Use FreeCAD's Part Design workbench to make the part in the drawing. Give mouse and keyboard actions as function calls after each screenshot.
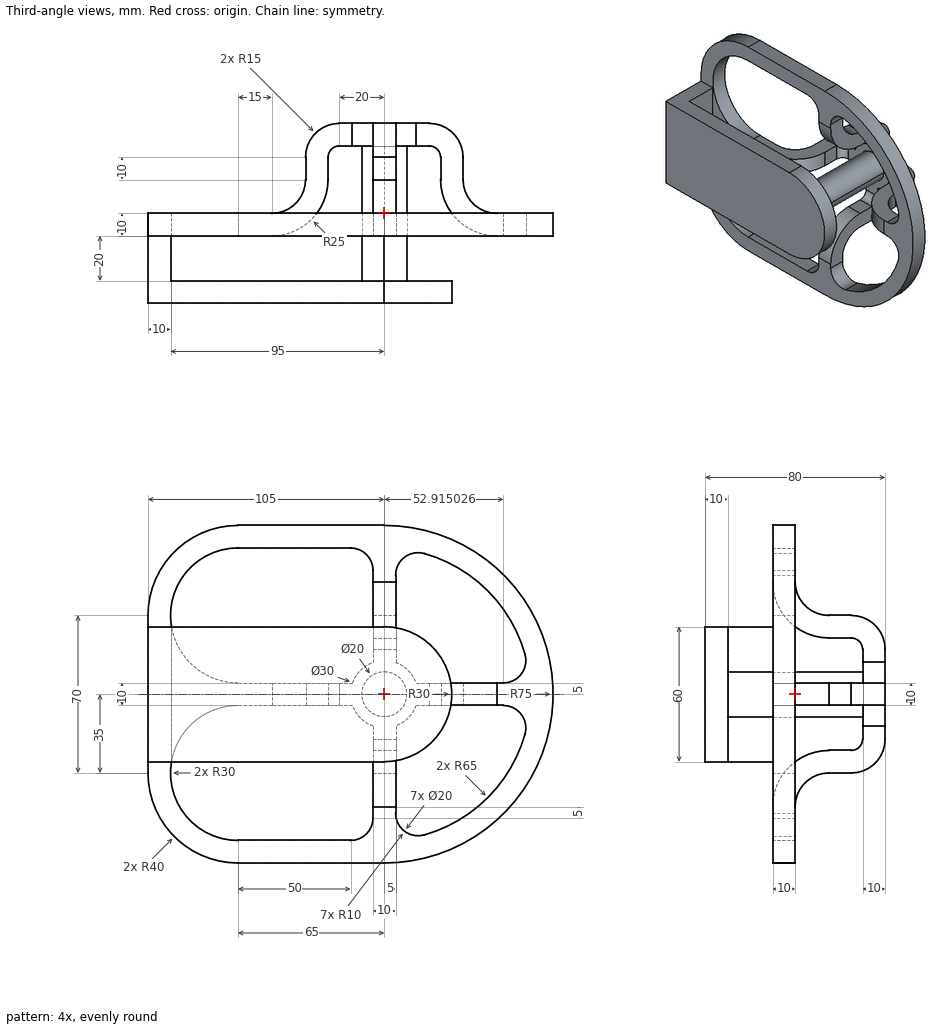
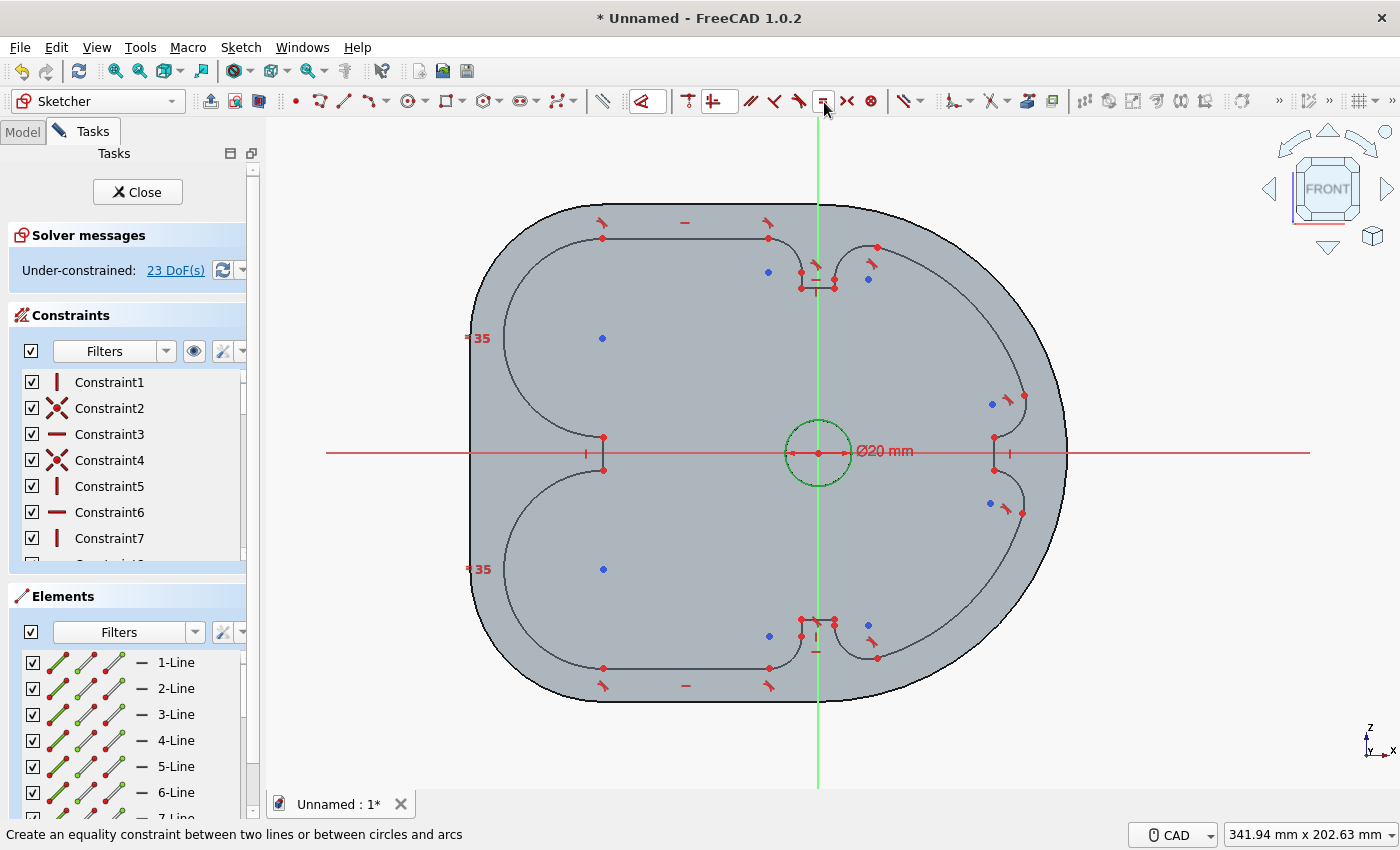
click(784, 665)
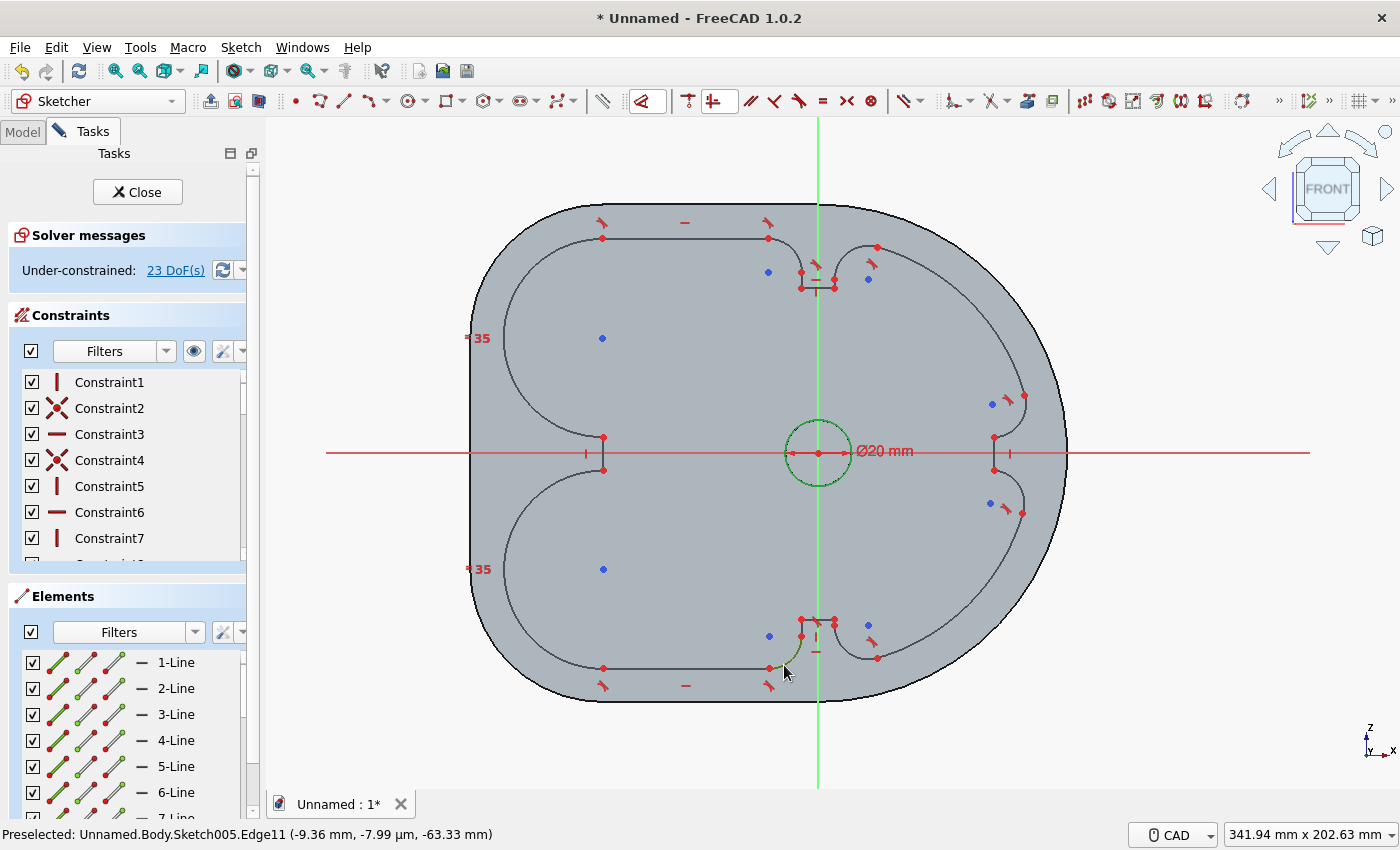
click(798, 257)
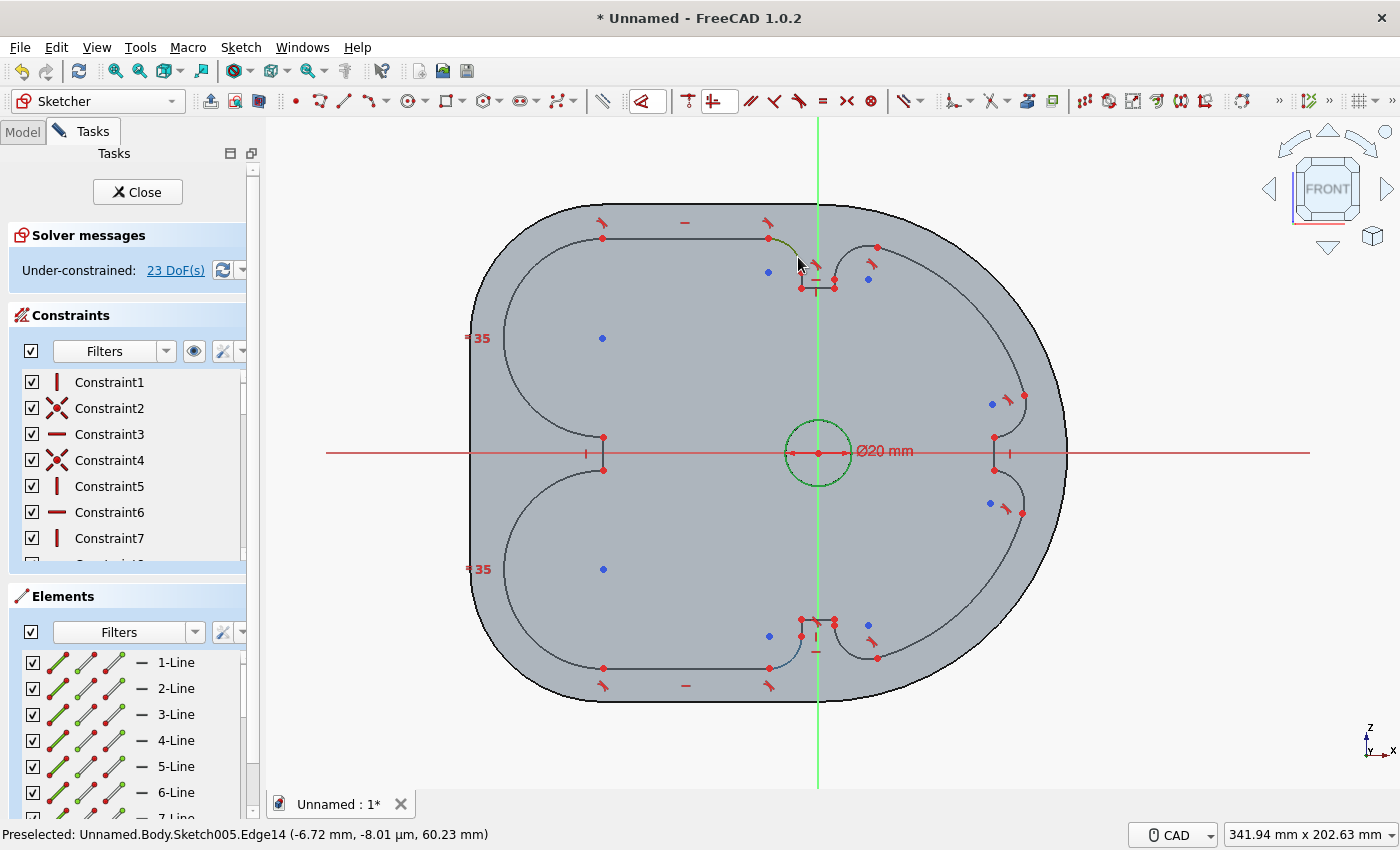
click(859, 247)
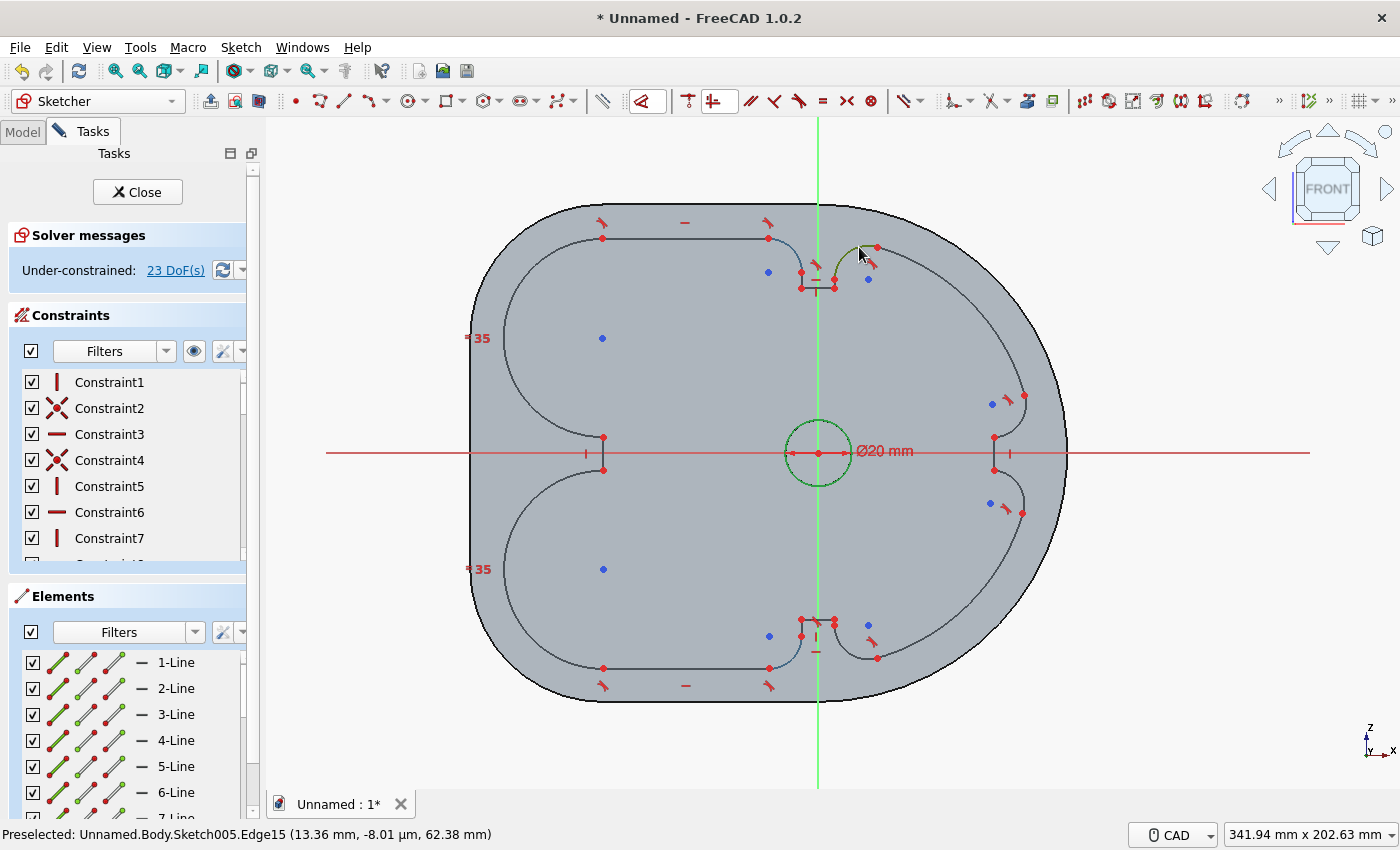
click(1011, 432)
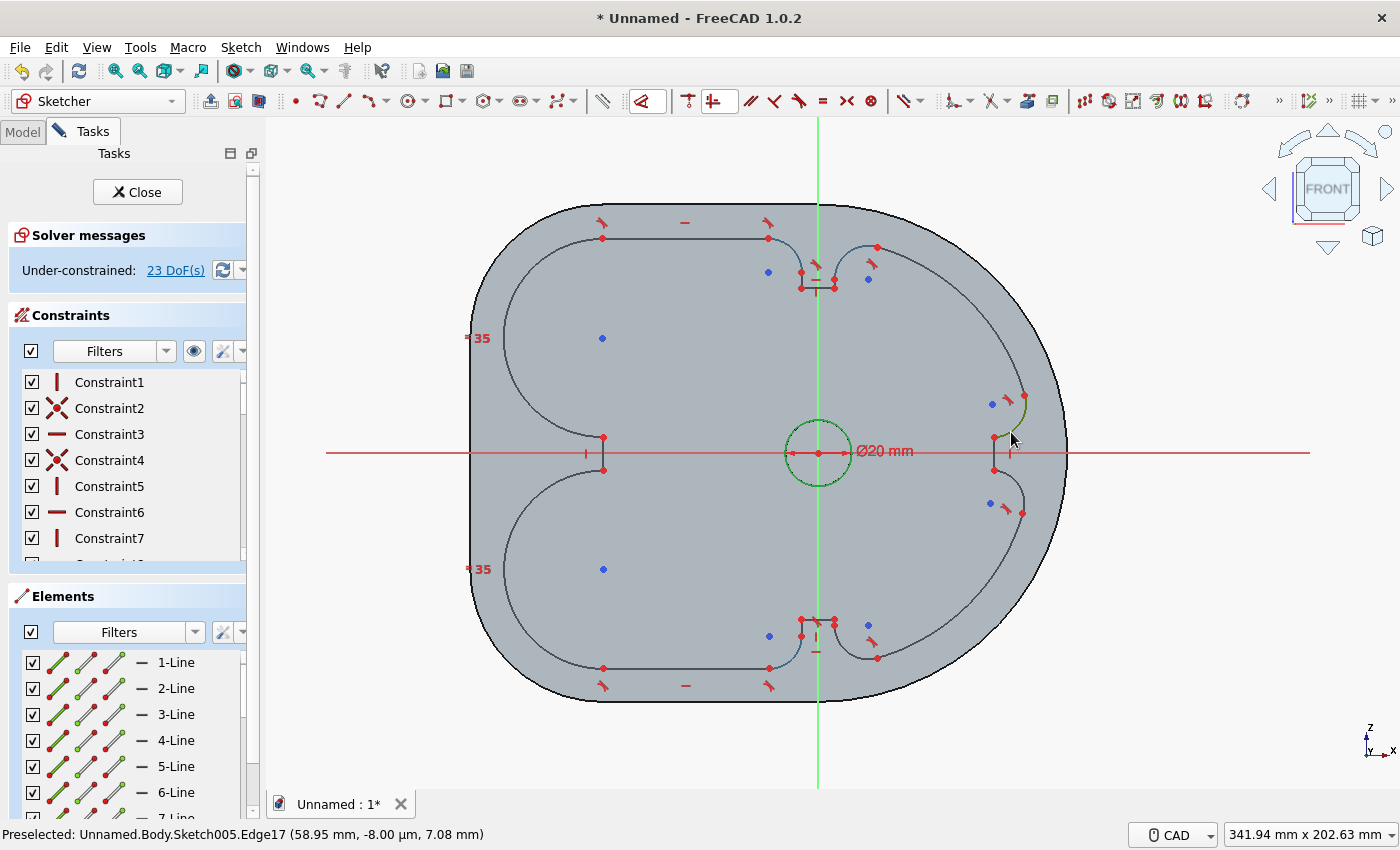
click(1023, 496)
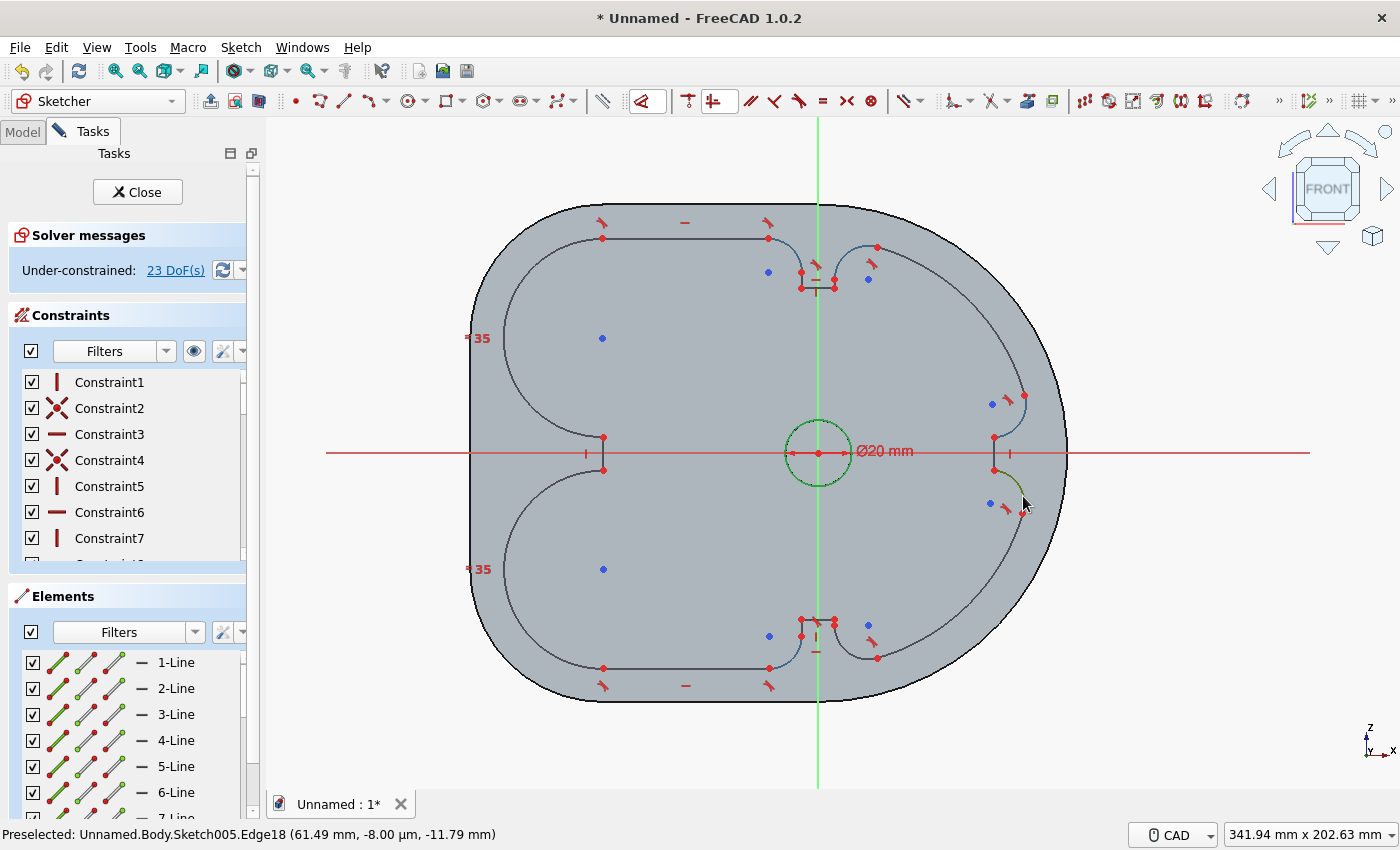
click(840, 644)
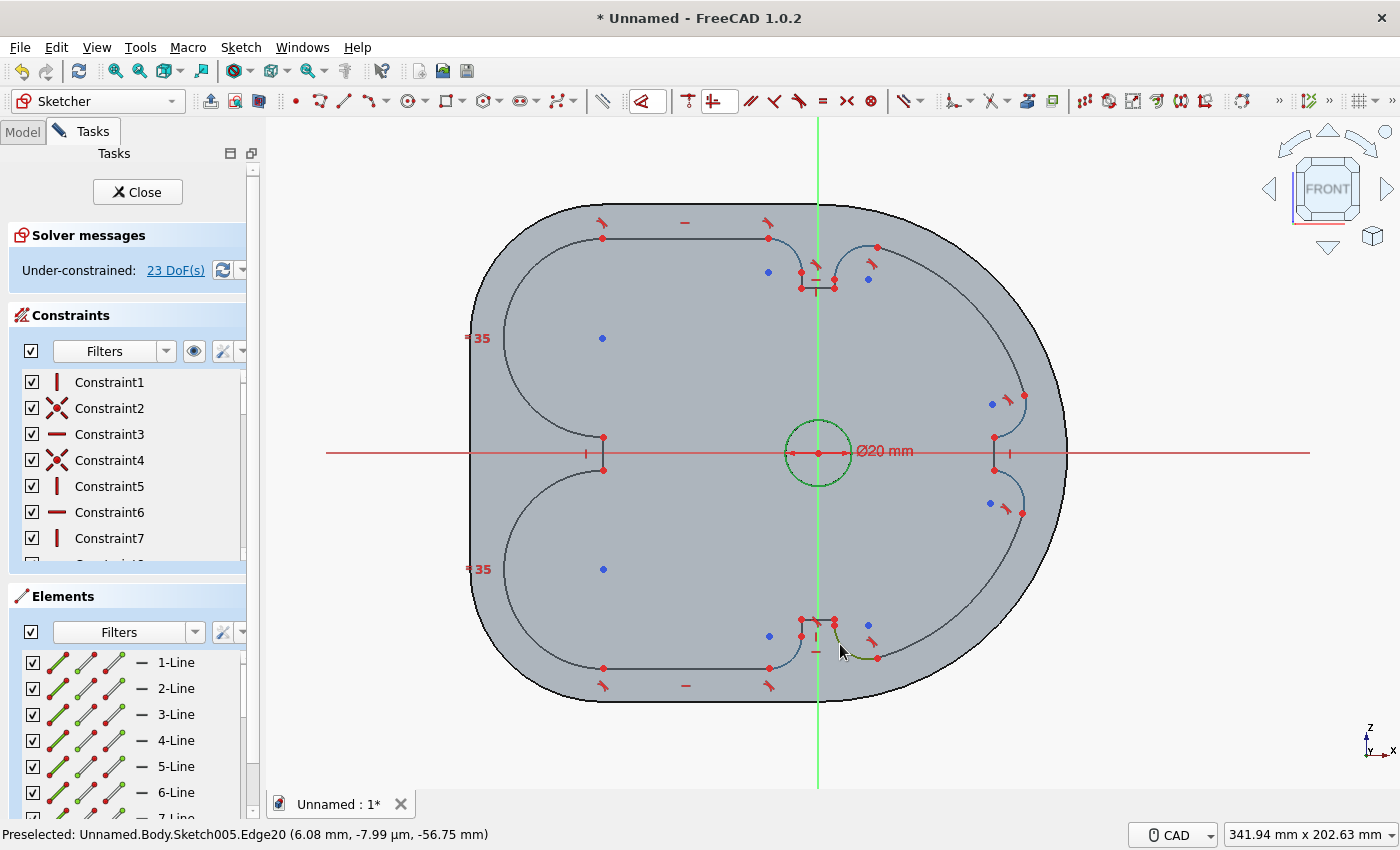
click(824, 102)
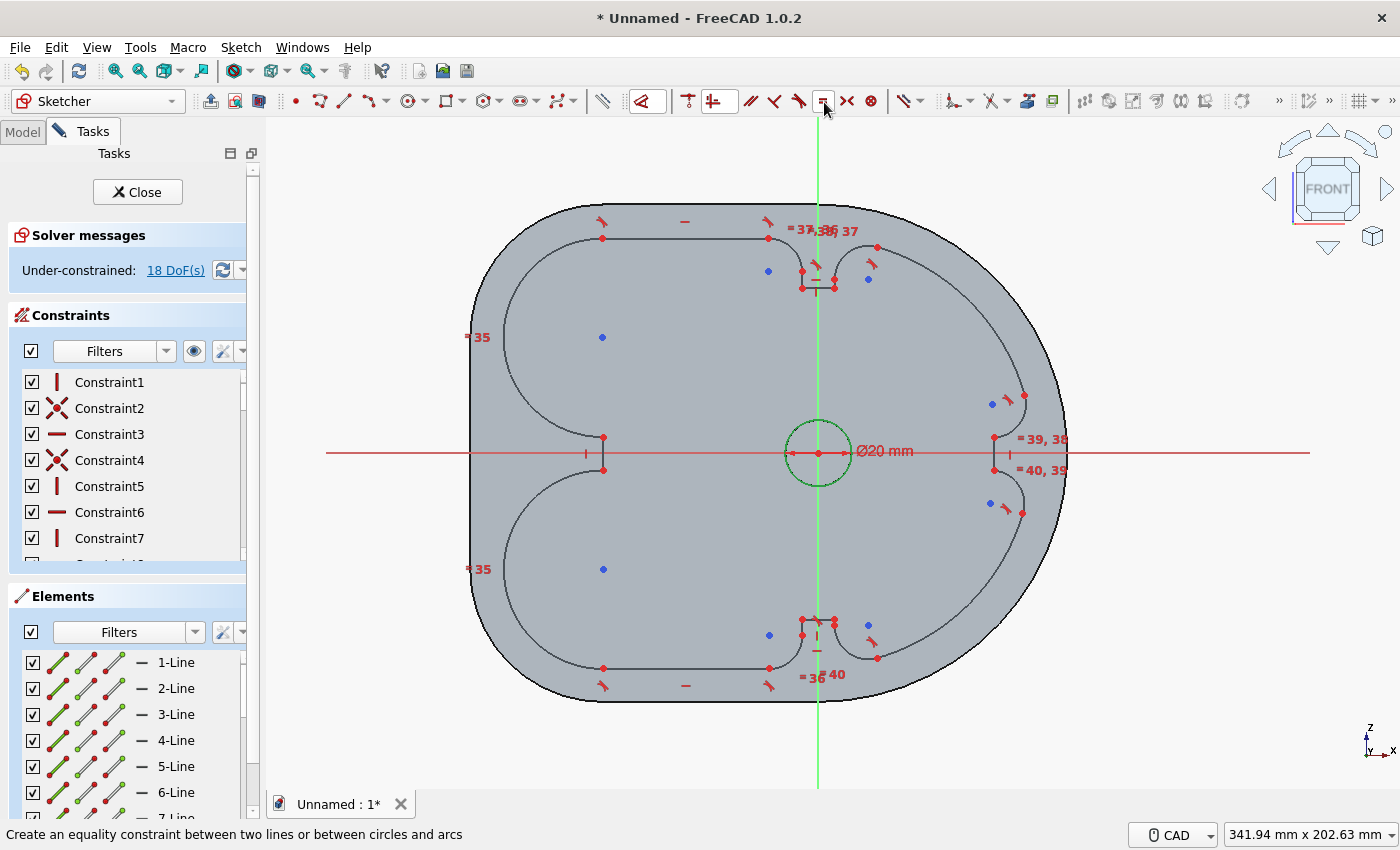
click(998, 336)